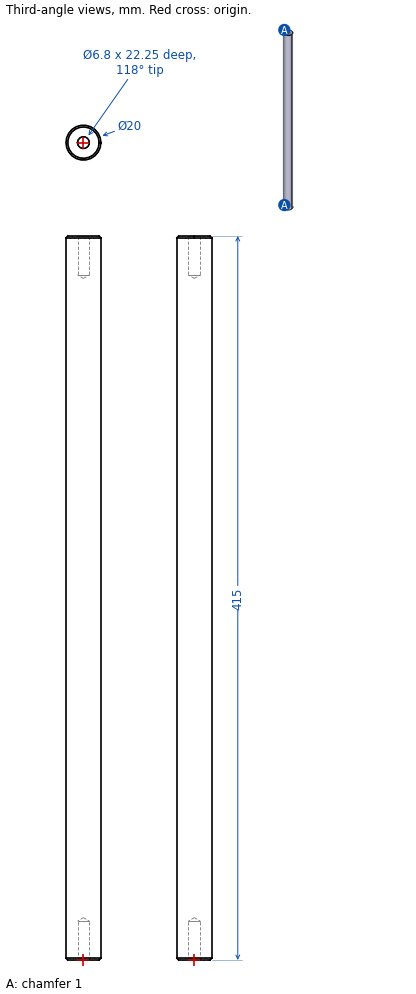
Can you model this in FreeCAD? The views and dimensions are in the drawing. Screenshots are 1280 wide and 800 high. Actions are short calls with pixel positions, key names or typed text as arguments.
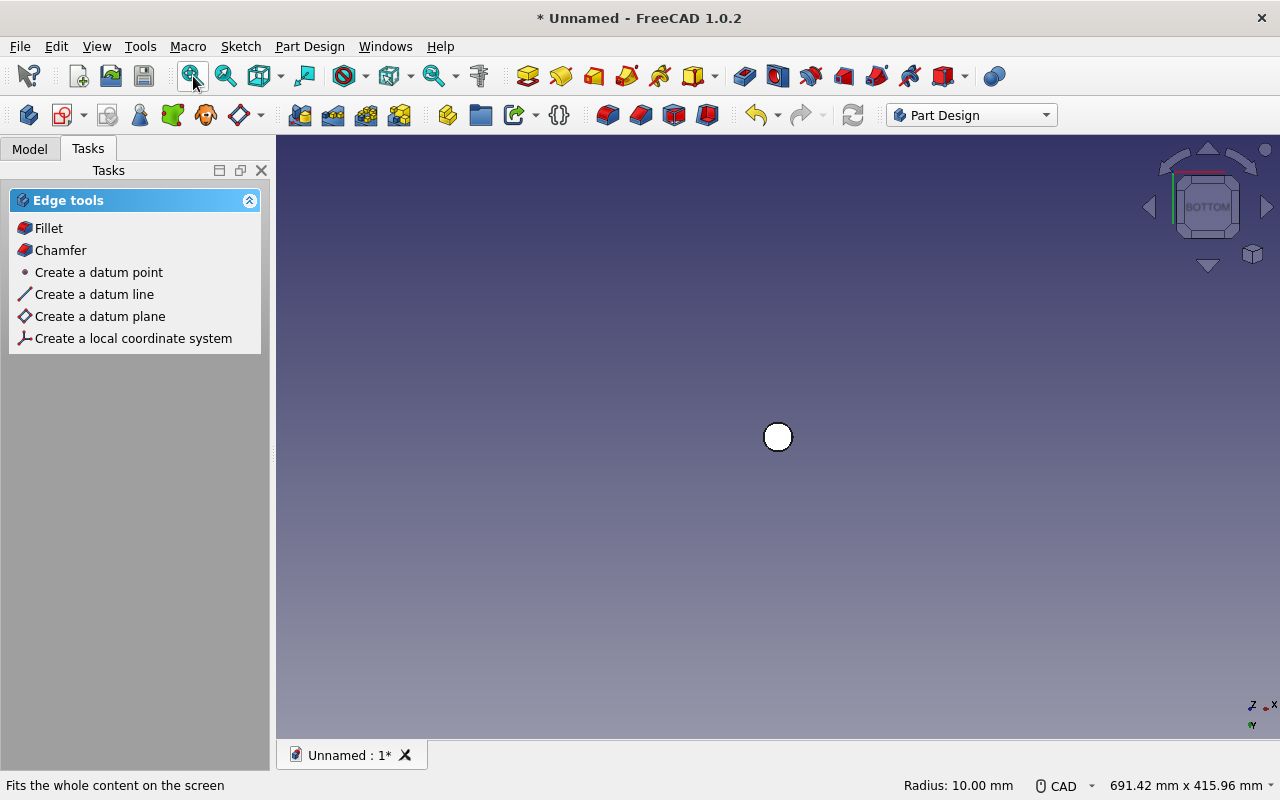
click(766, 445, ctrl)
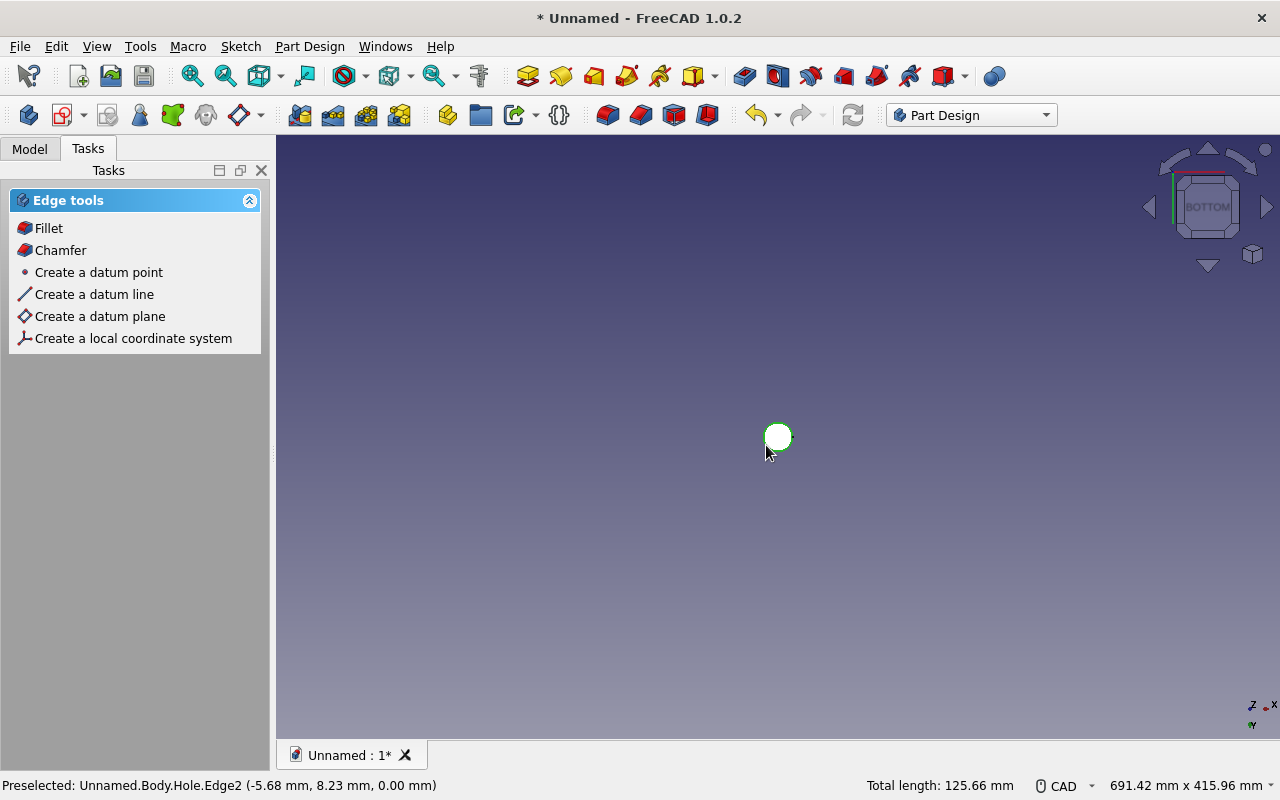
click(641, 116)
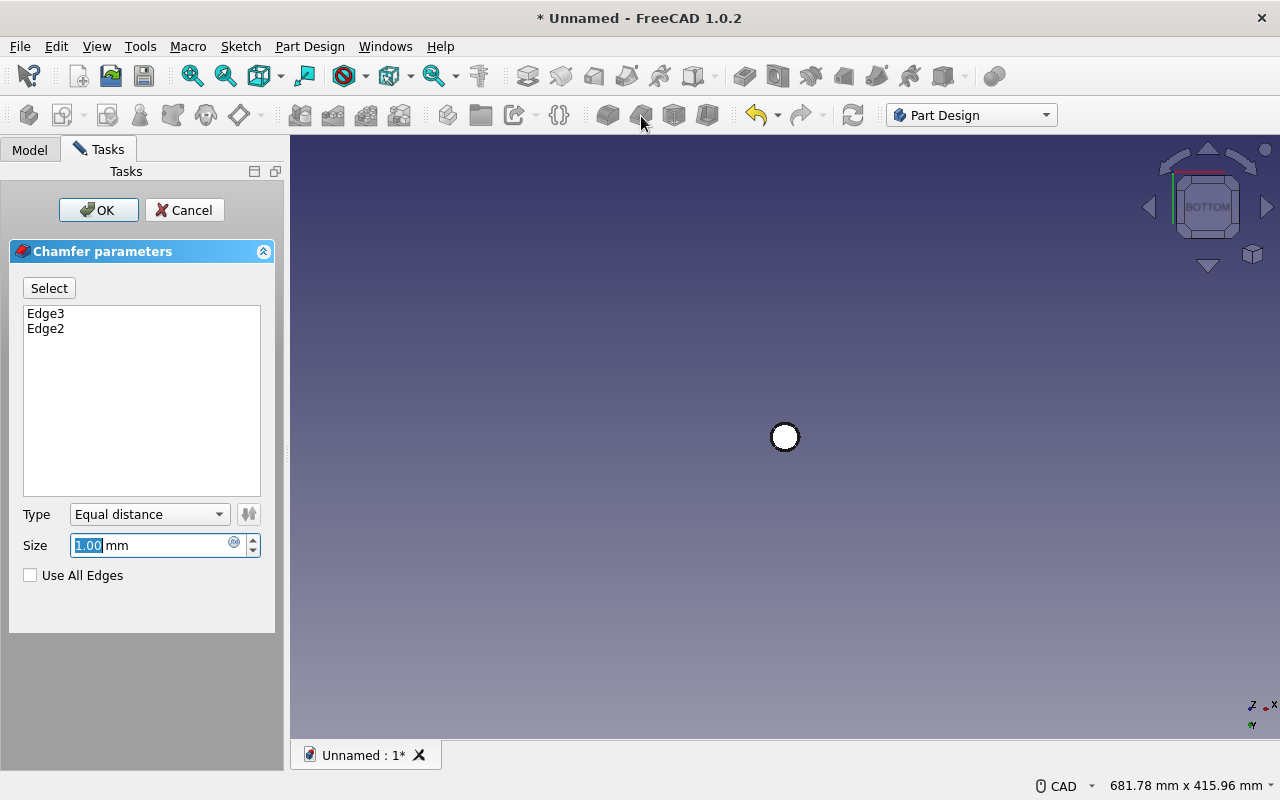
text(1)
key(Tab)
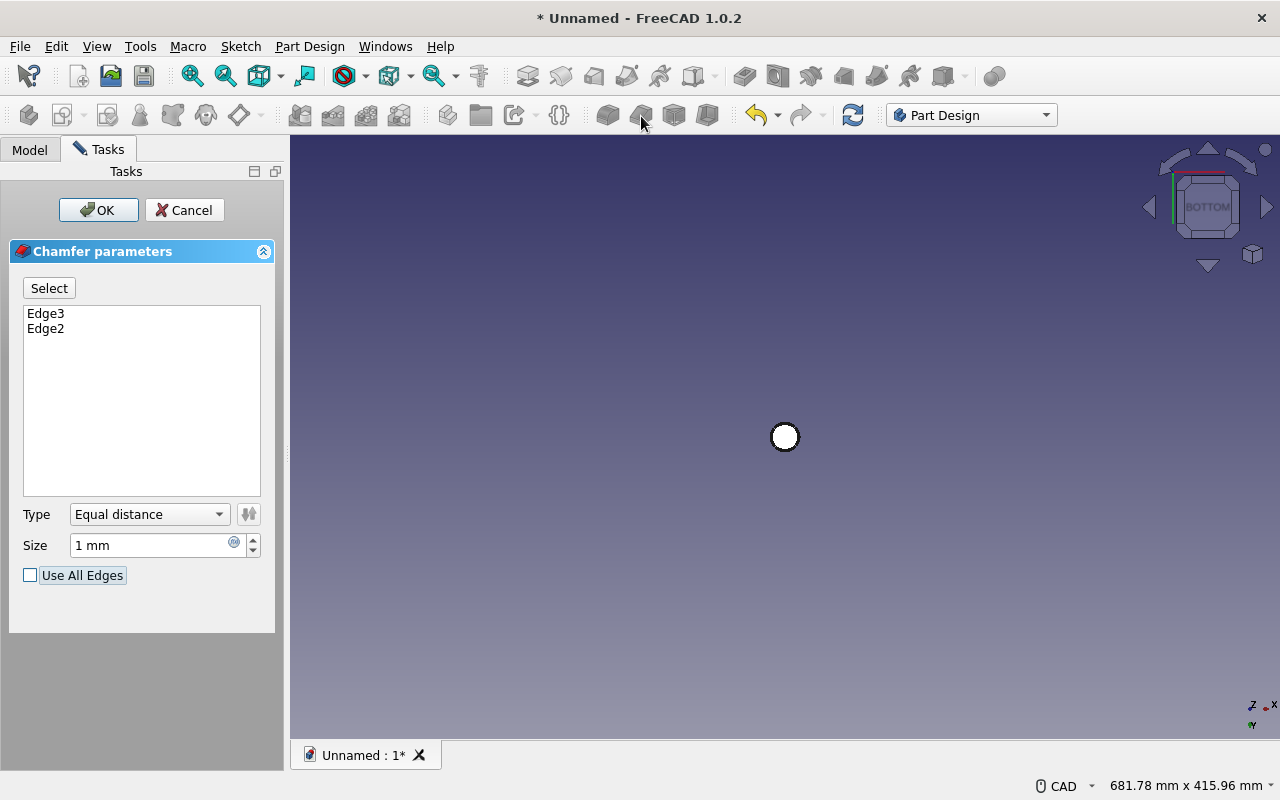
click(99, 210)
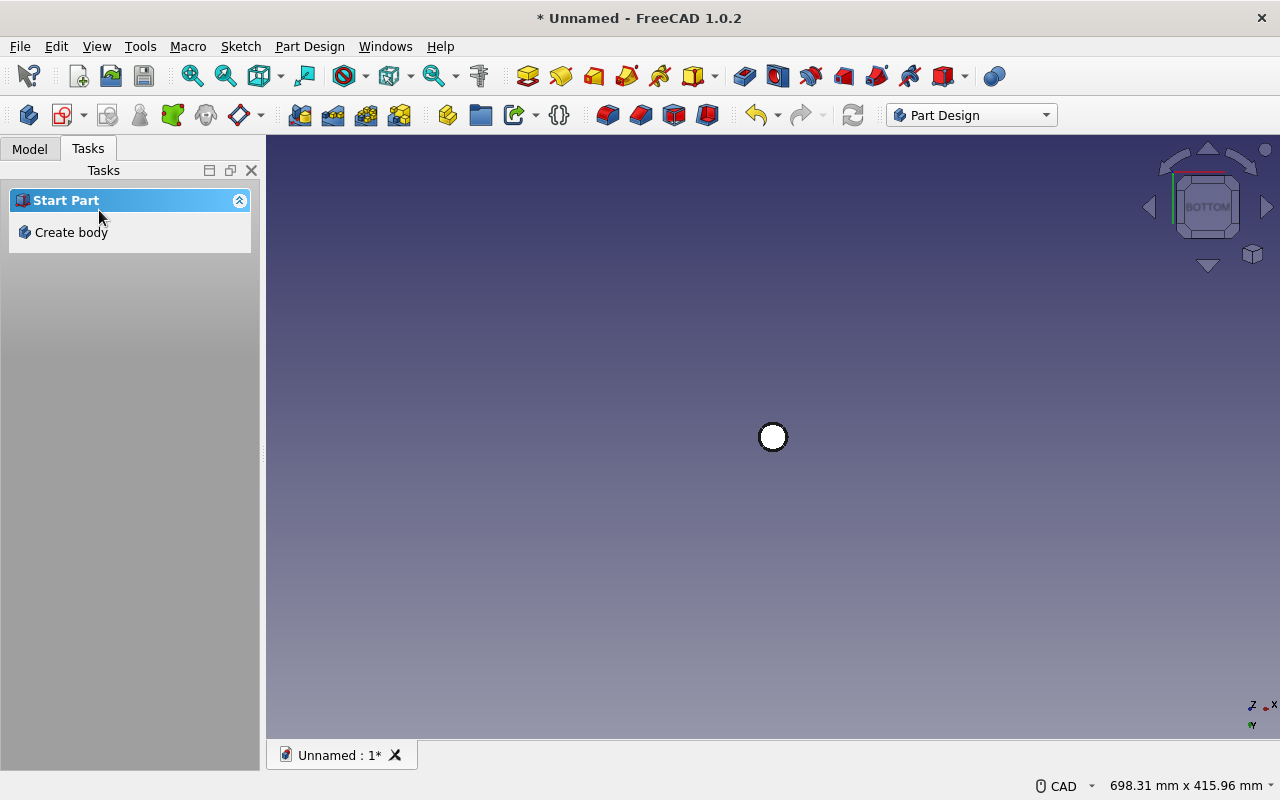
click(193, 76)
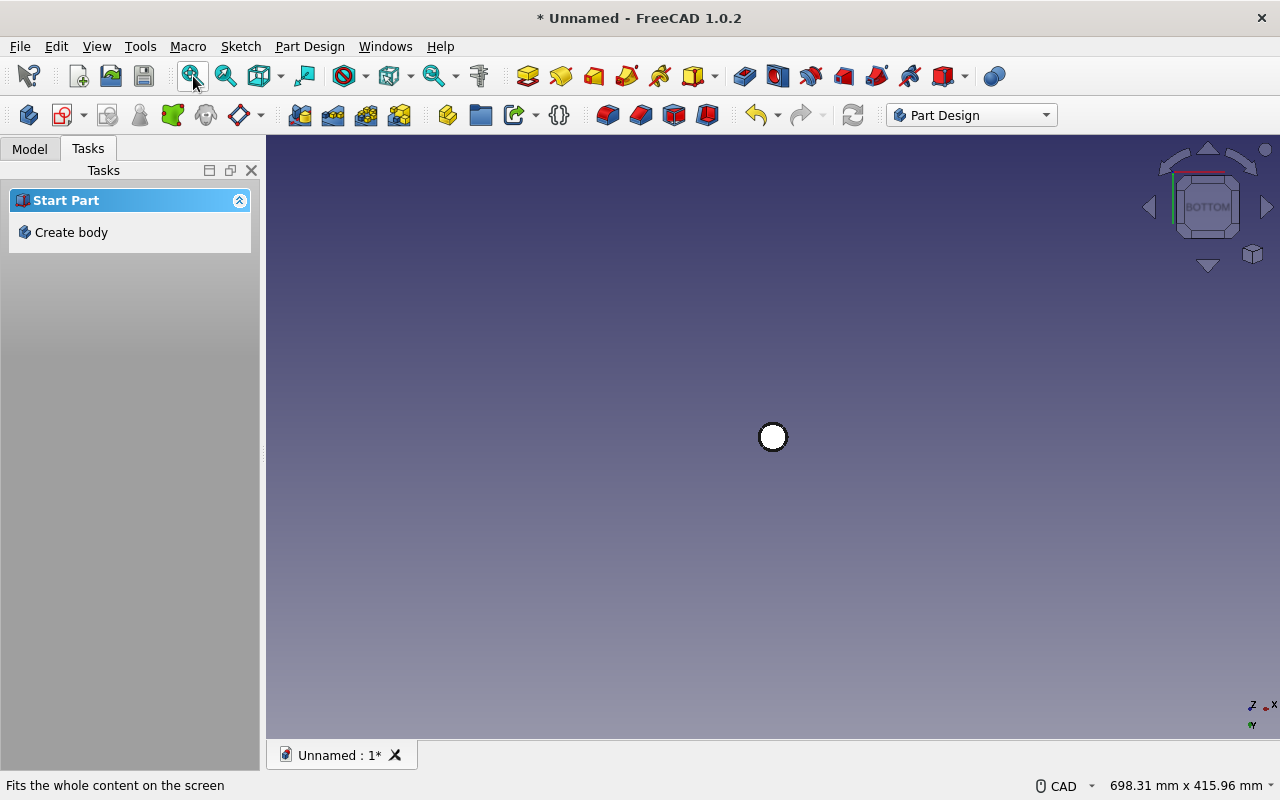
click(773, 436)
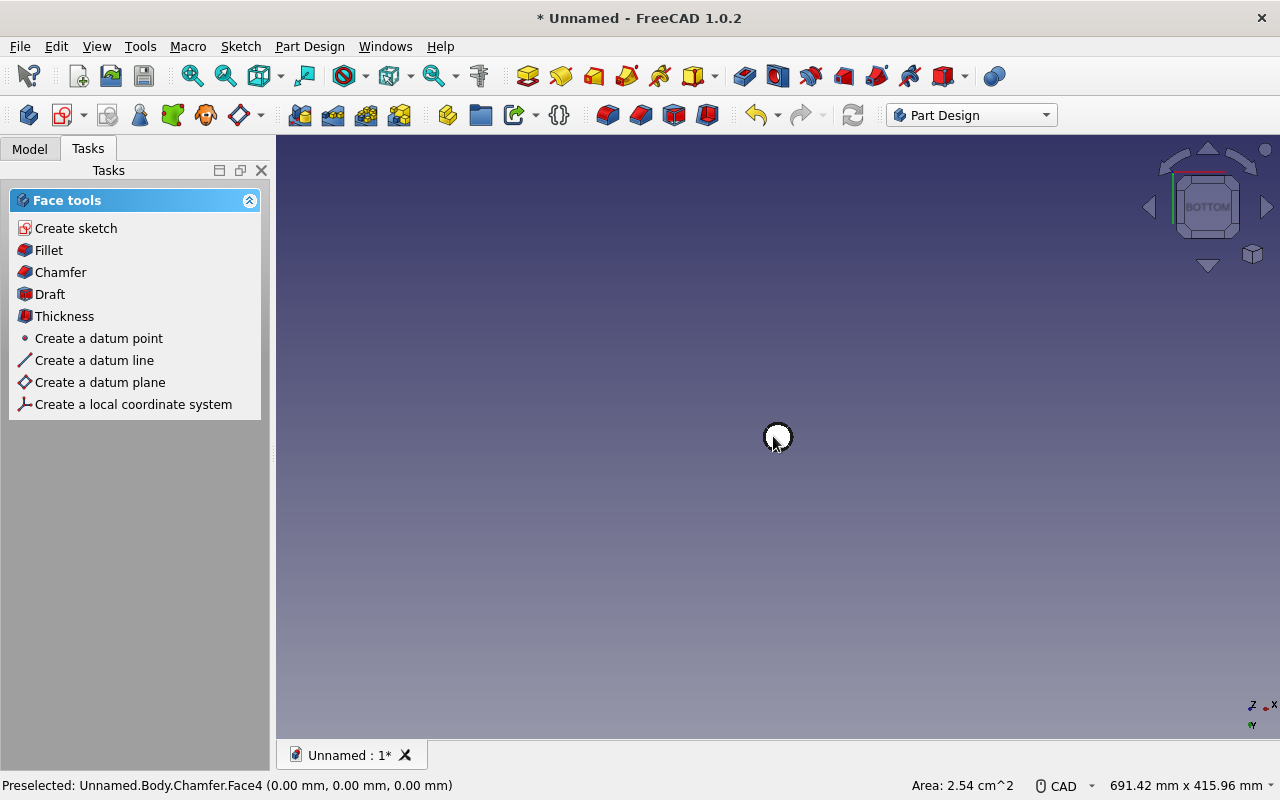
click(62, 116)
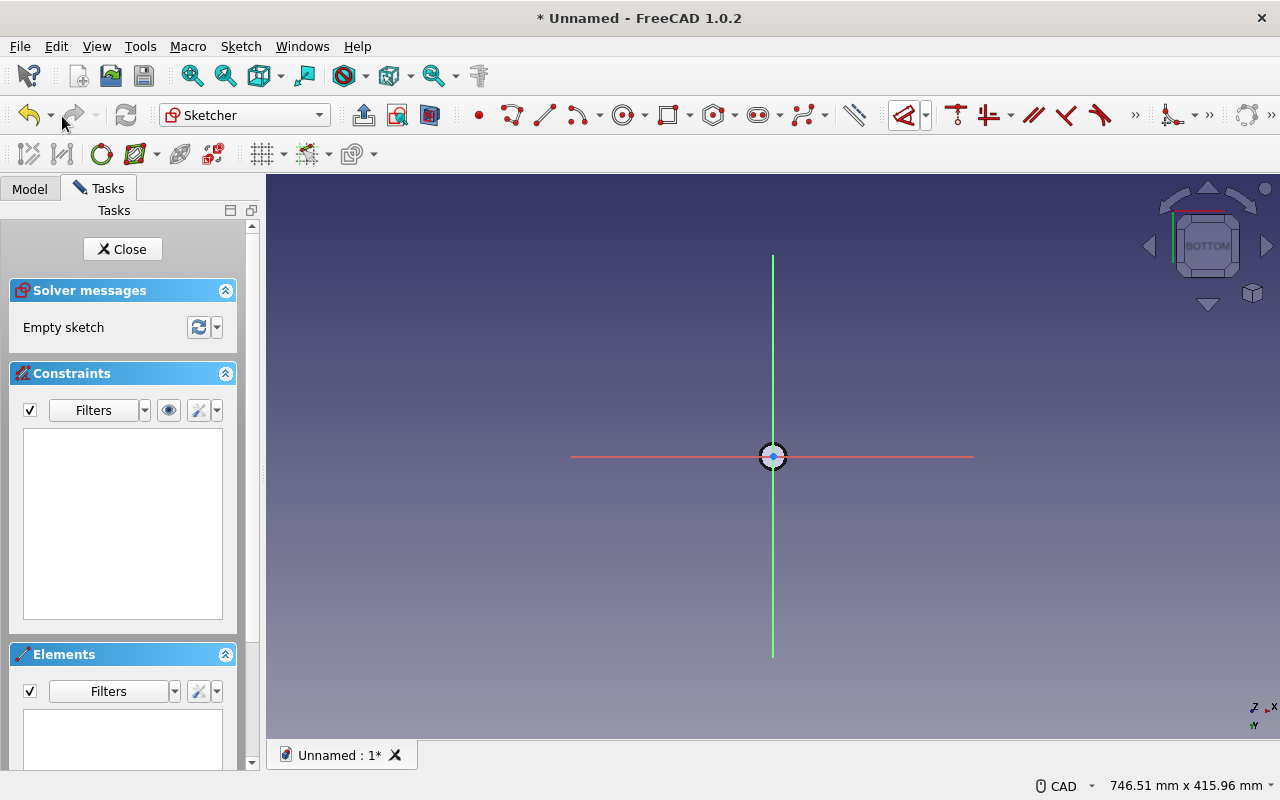
scroll(777, 457, up, 15)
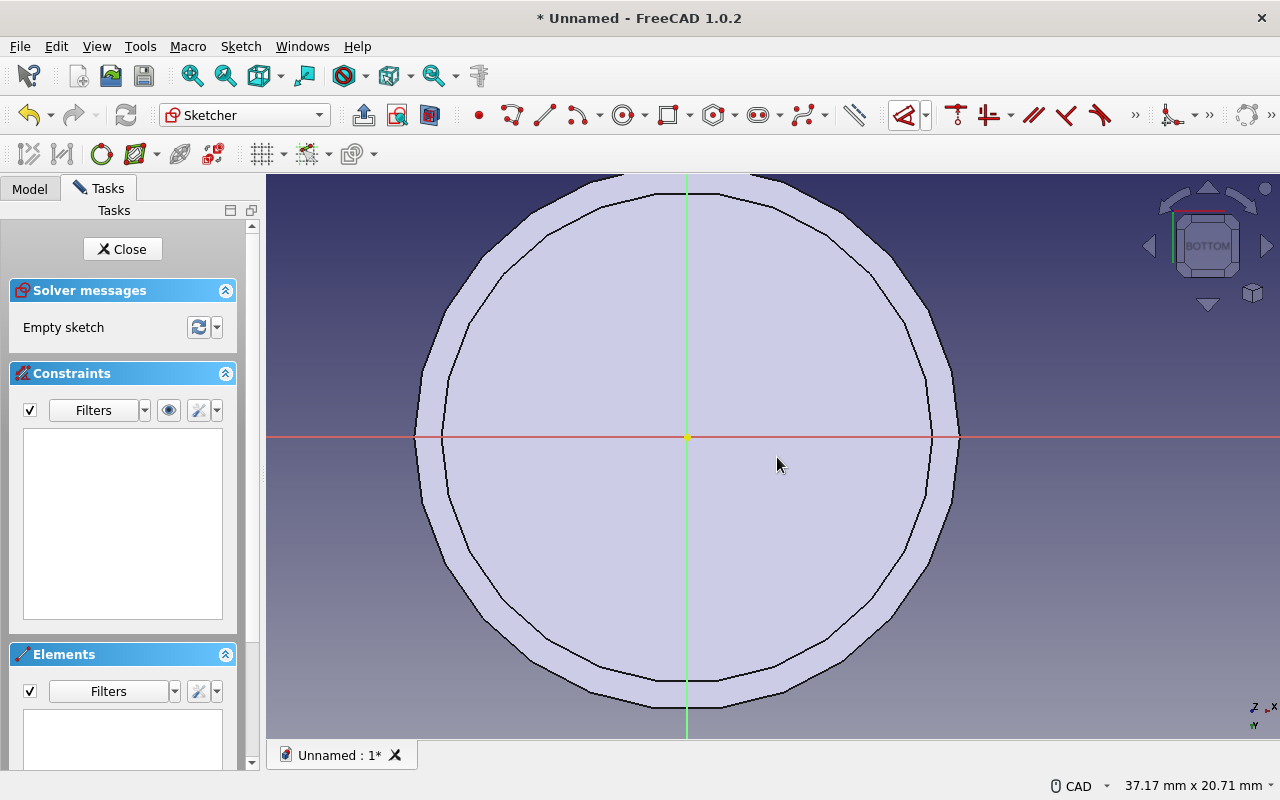
scroll(666, 414, up, 3)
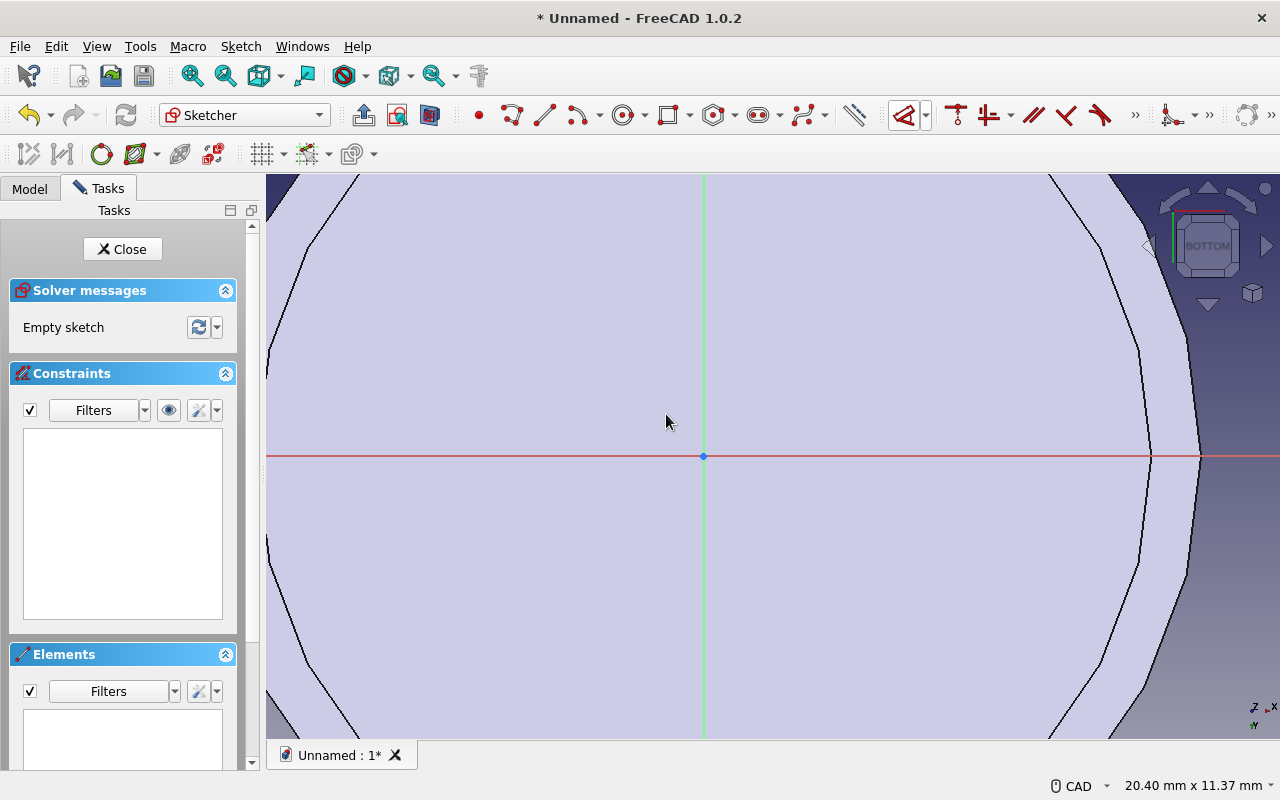
click(622, 116)